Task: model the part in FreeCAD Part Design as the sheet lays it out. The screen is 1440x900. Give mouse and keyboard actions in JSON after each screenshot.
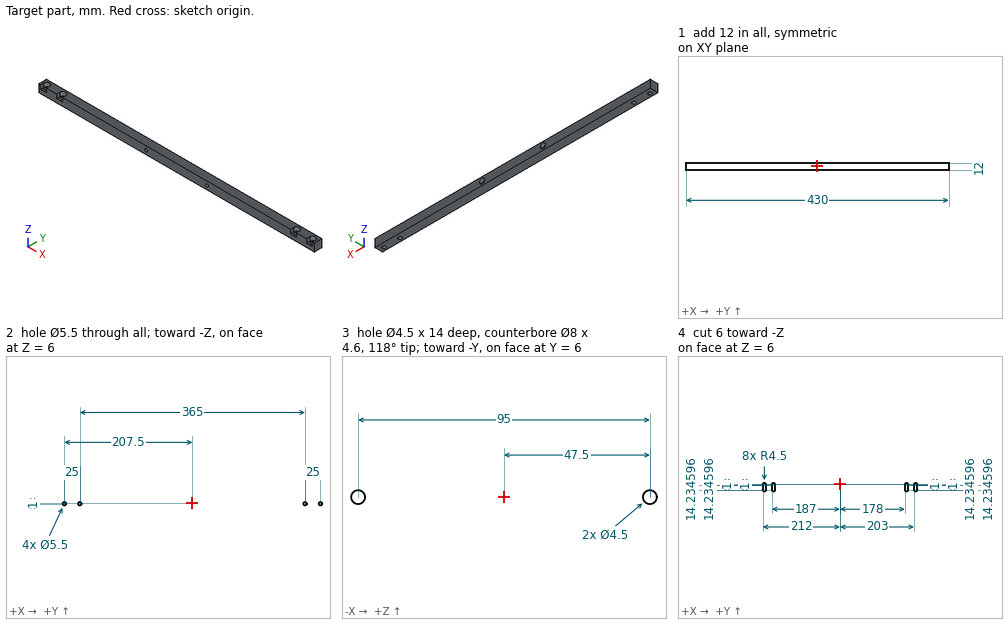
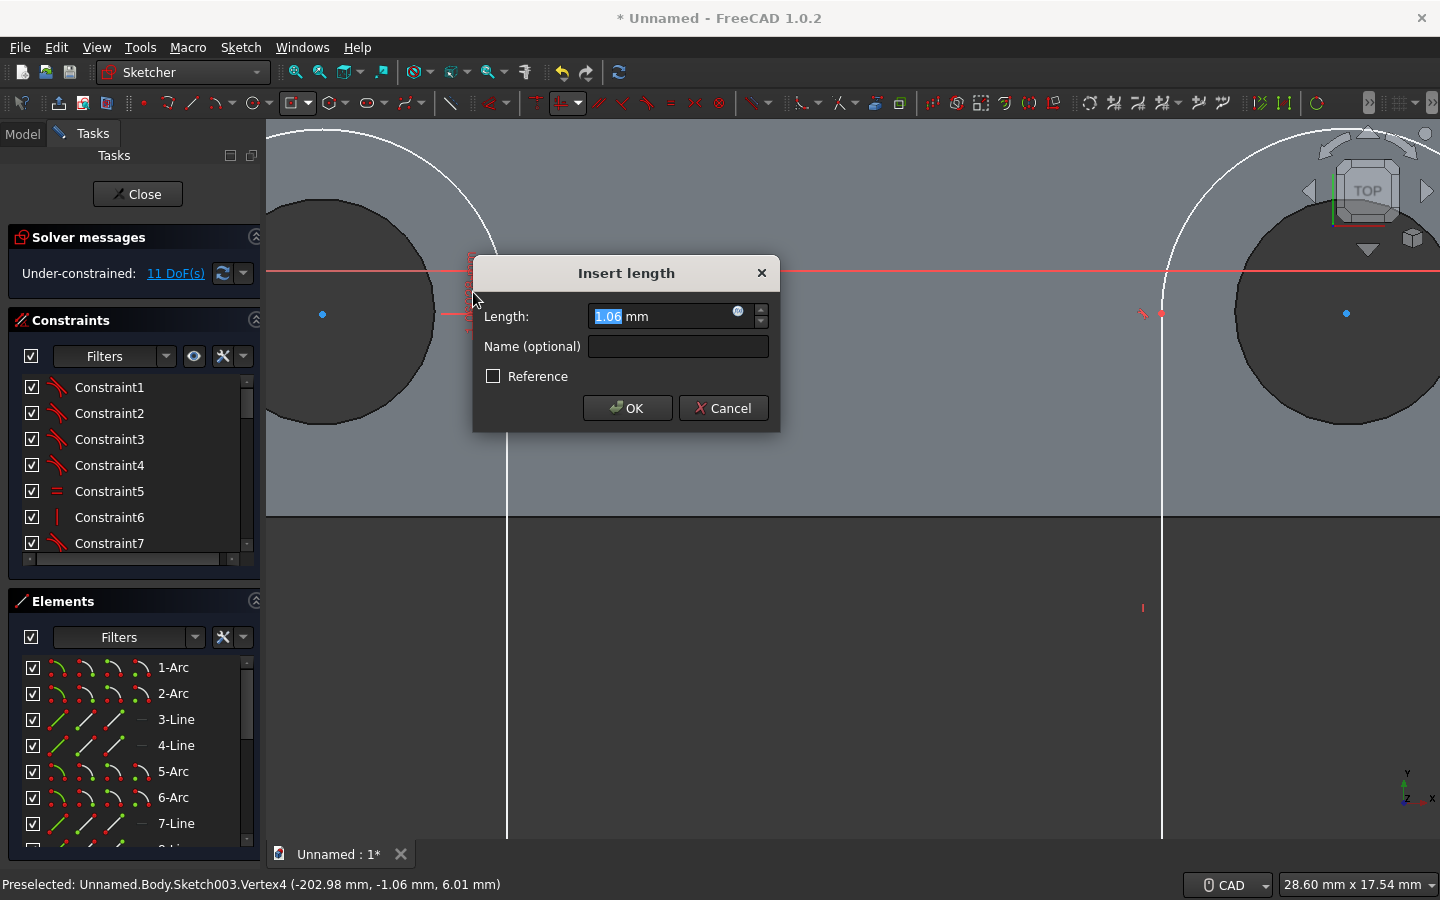
{"action": "type", "text": "1"}
{"action": "key", "text": "Return"}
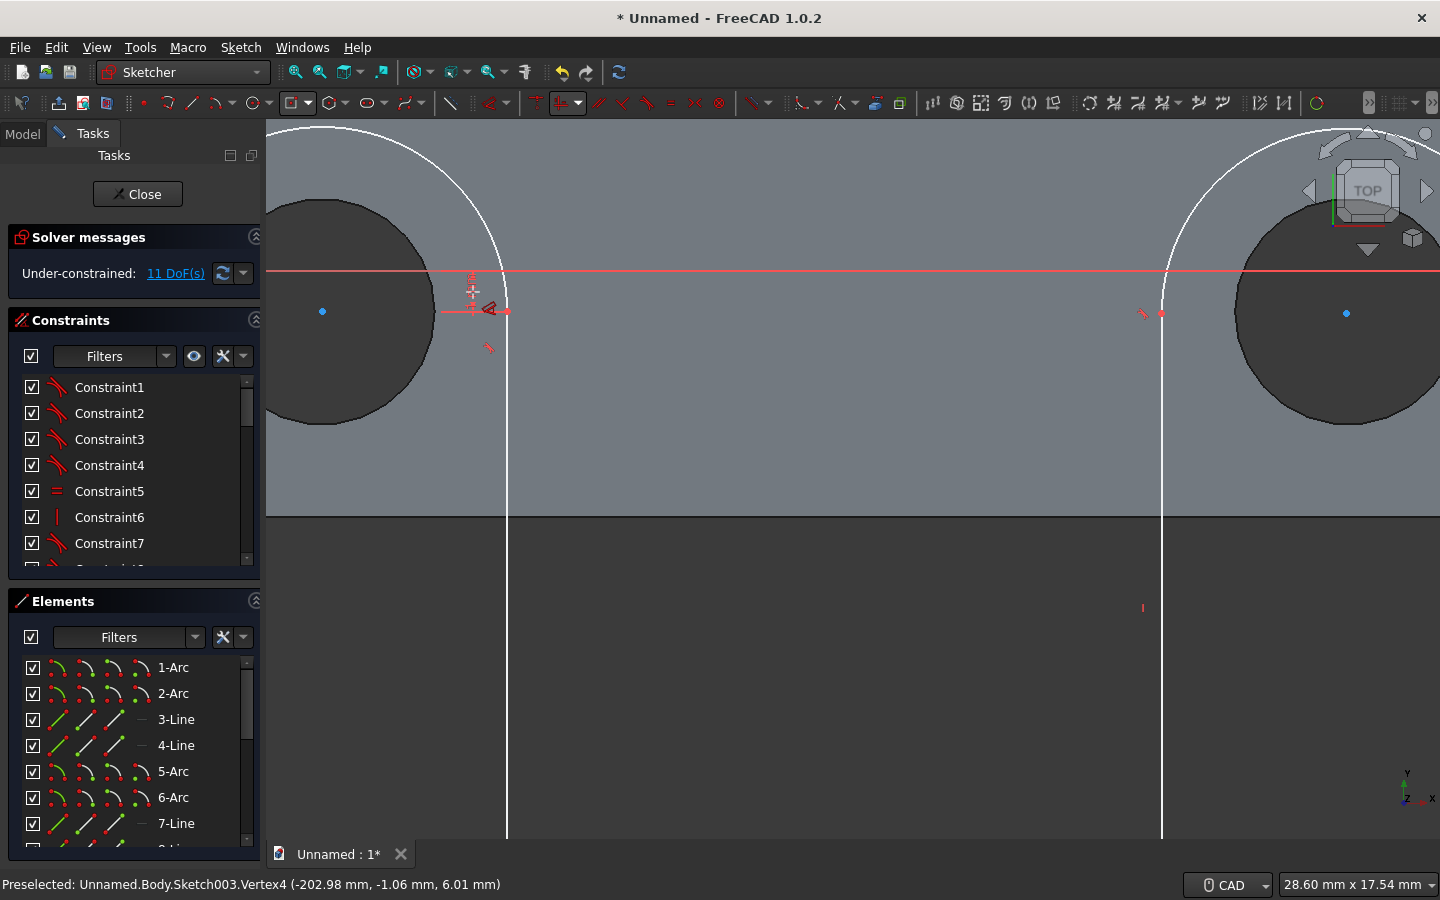
{"action": "scroll", "coordinate": [362, 472], "scroll_direction": "down", "scroll_amount": 15}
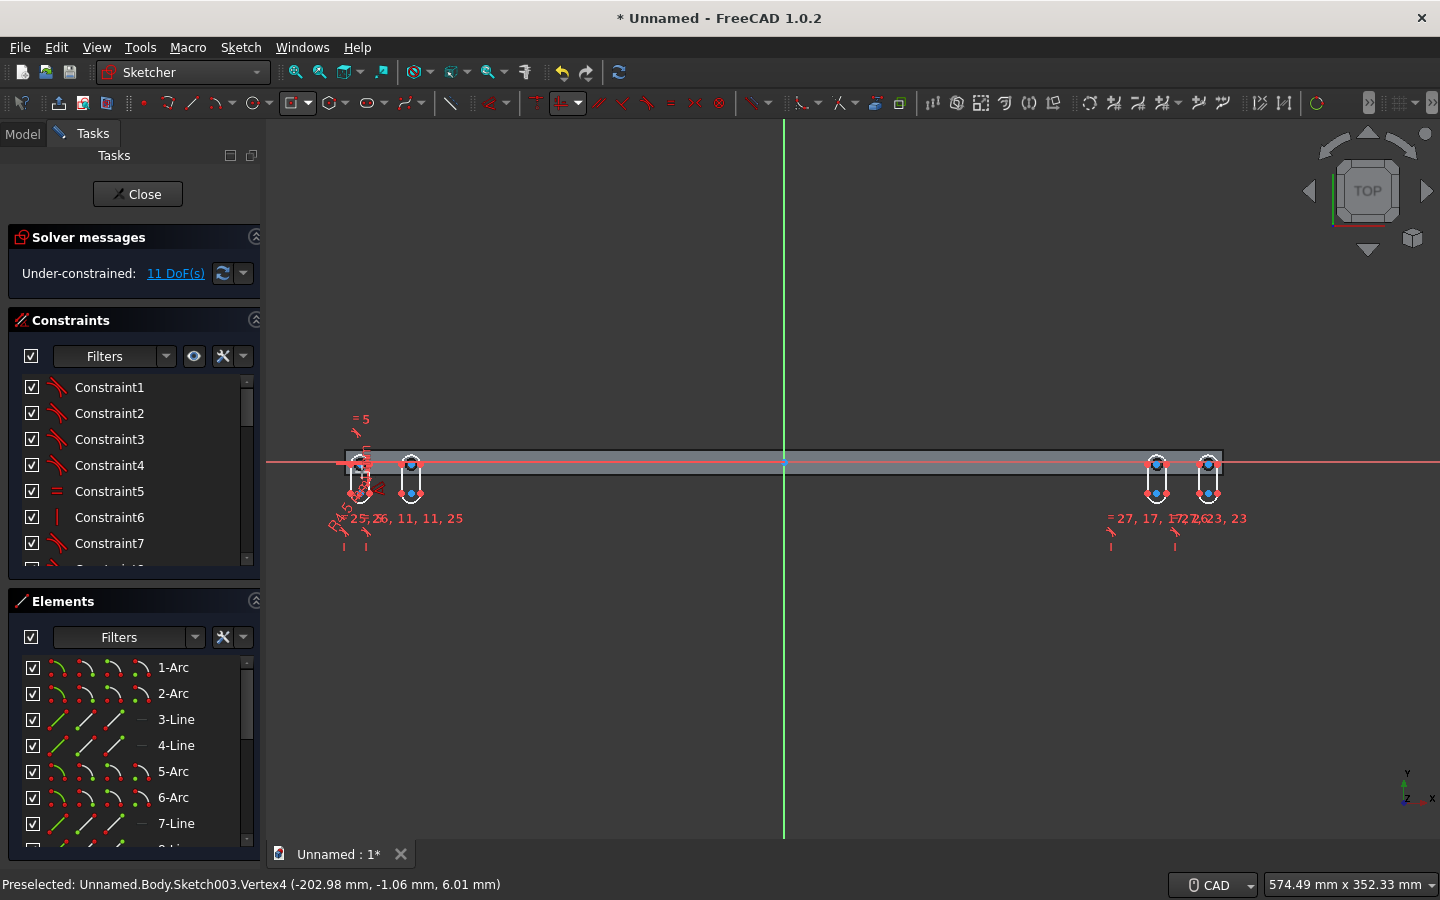
{"action": "scroll", "coordinate": [420, 465], "scroll_direction": "up", "scroll_amount": 15}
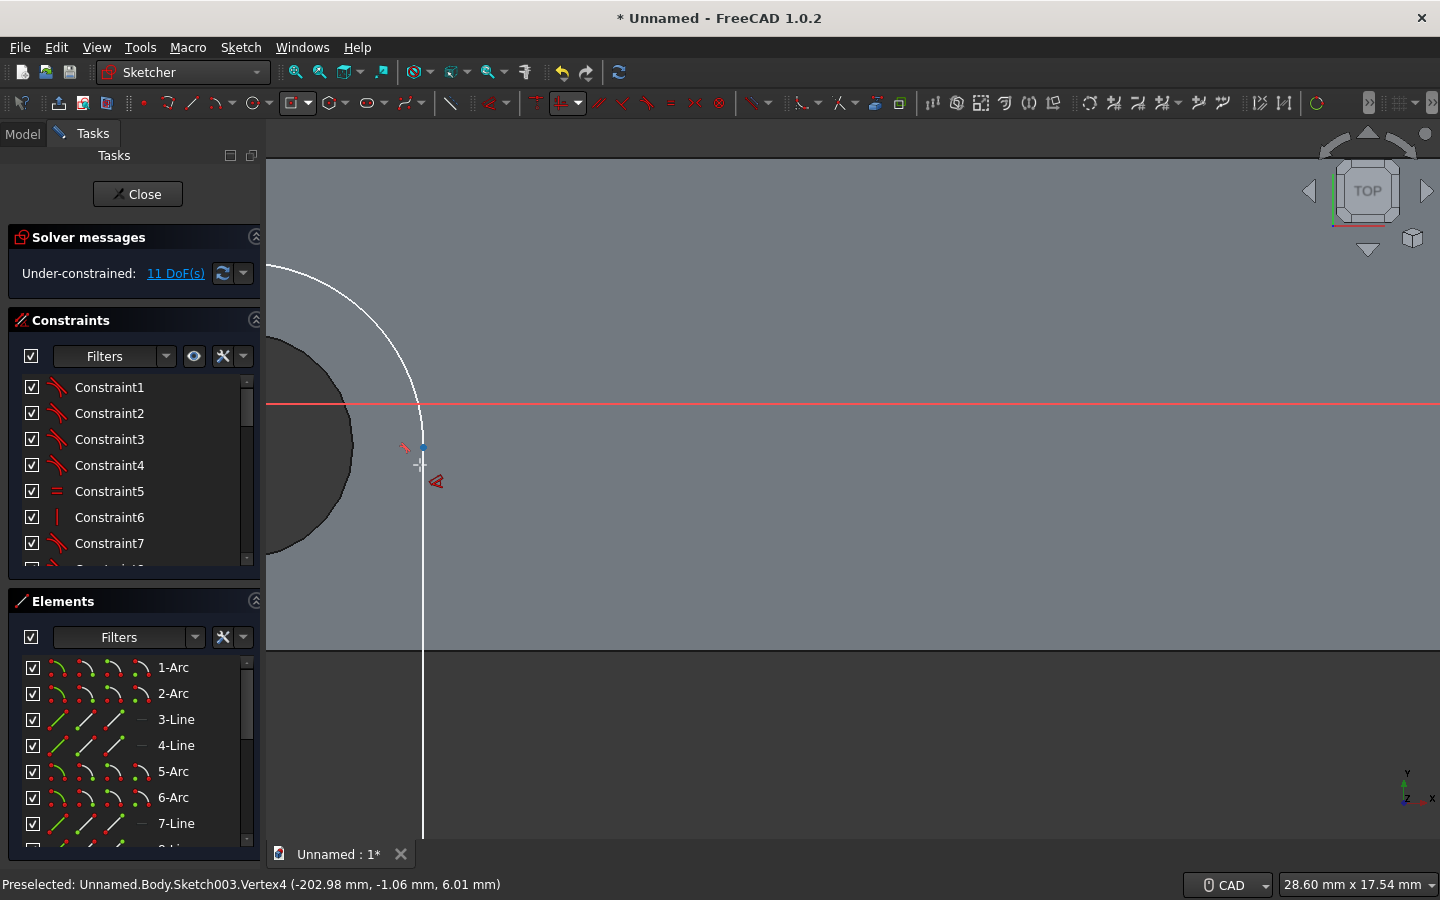
{"action": "left_click", "coordinate": [423, 447]}
{"action": "left_click", "coordinate": [389, 426]}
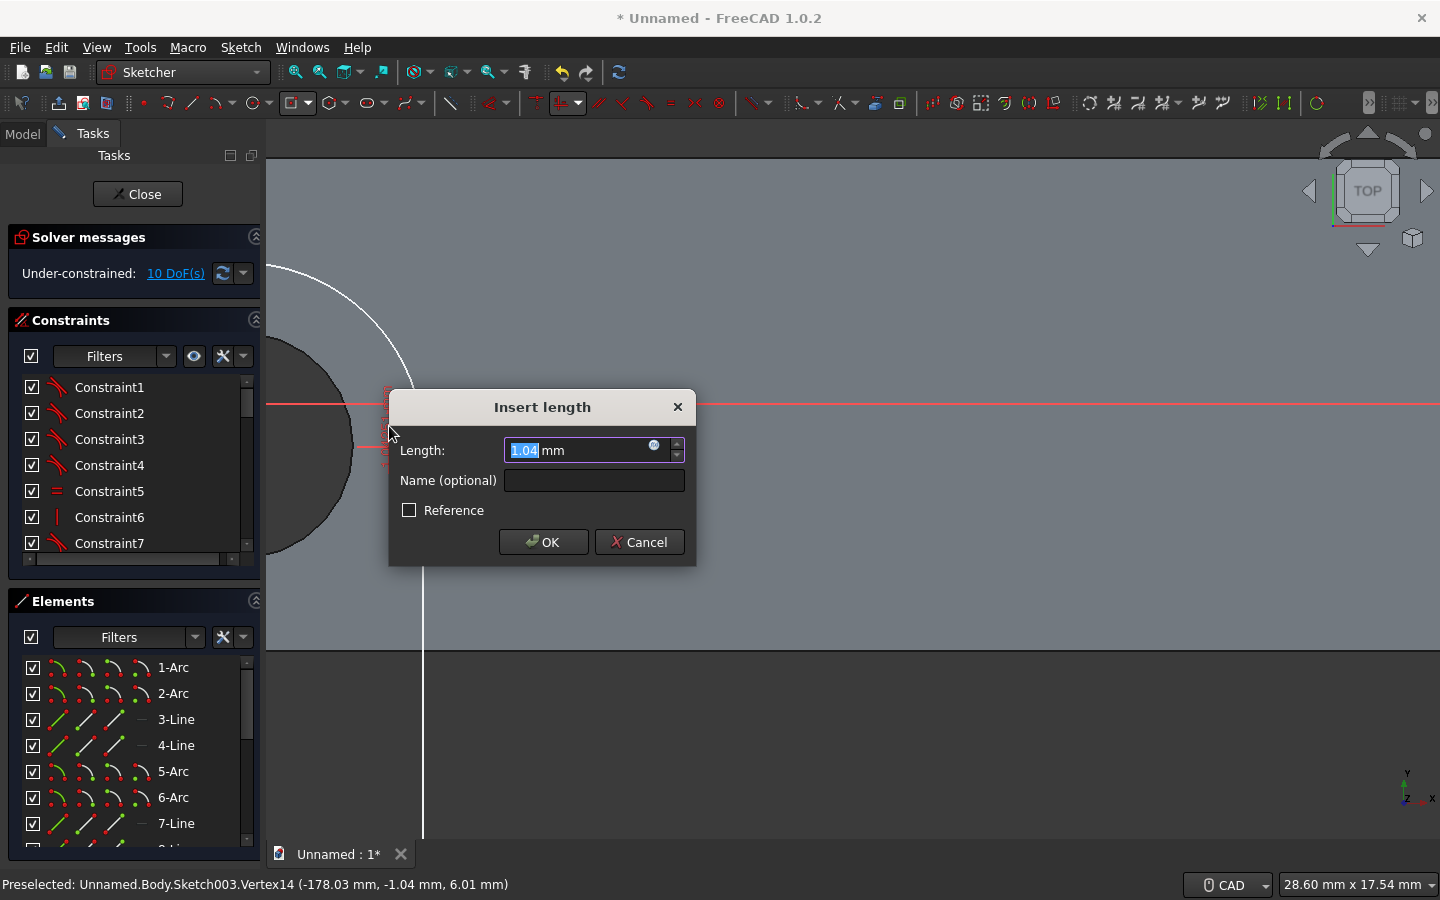
{"action": "type", "text": "1"}
{"action": "key", "text": "Return"}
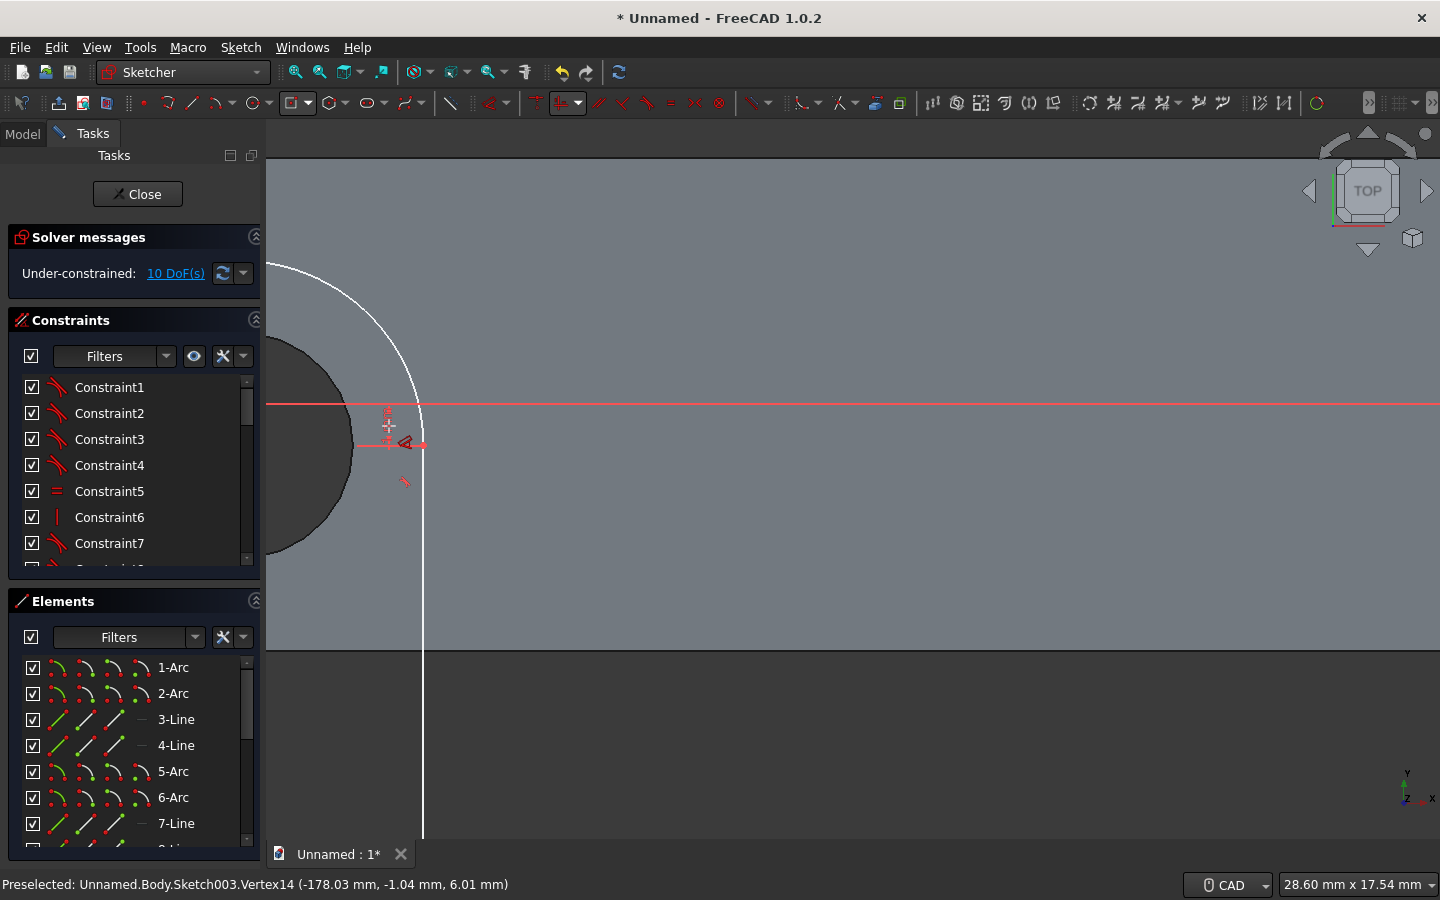
{"action": "scroll", "coordinate": [421, 465], "scroll_direction": "down", "scroll_amount": 15}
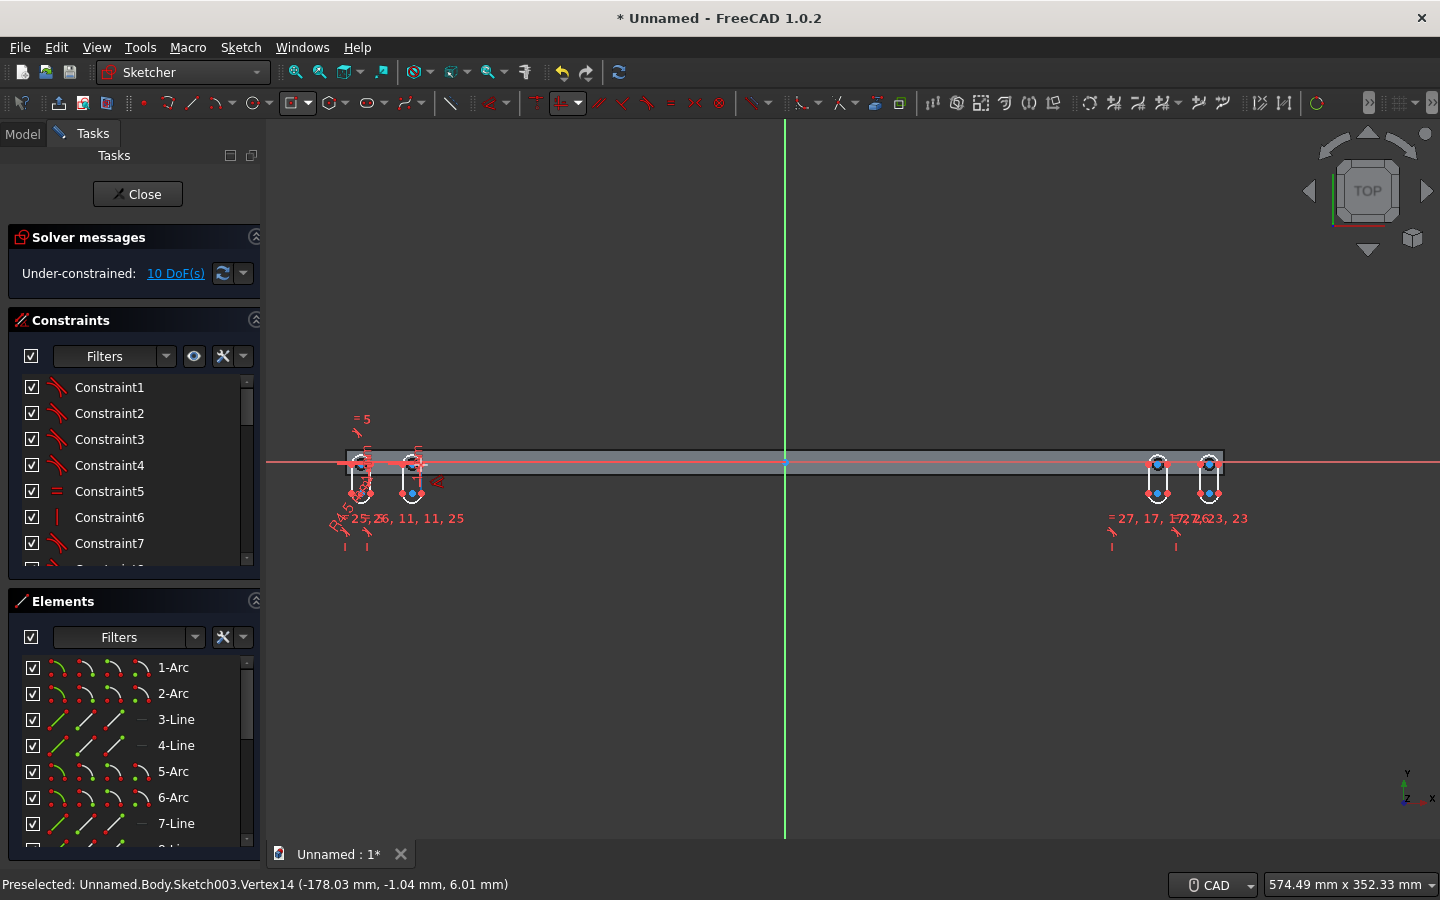
{"action": "scroll", "coordinate": [1167, 465], "scroll_direction": "up", "scroll_amount": 15}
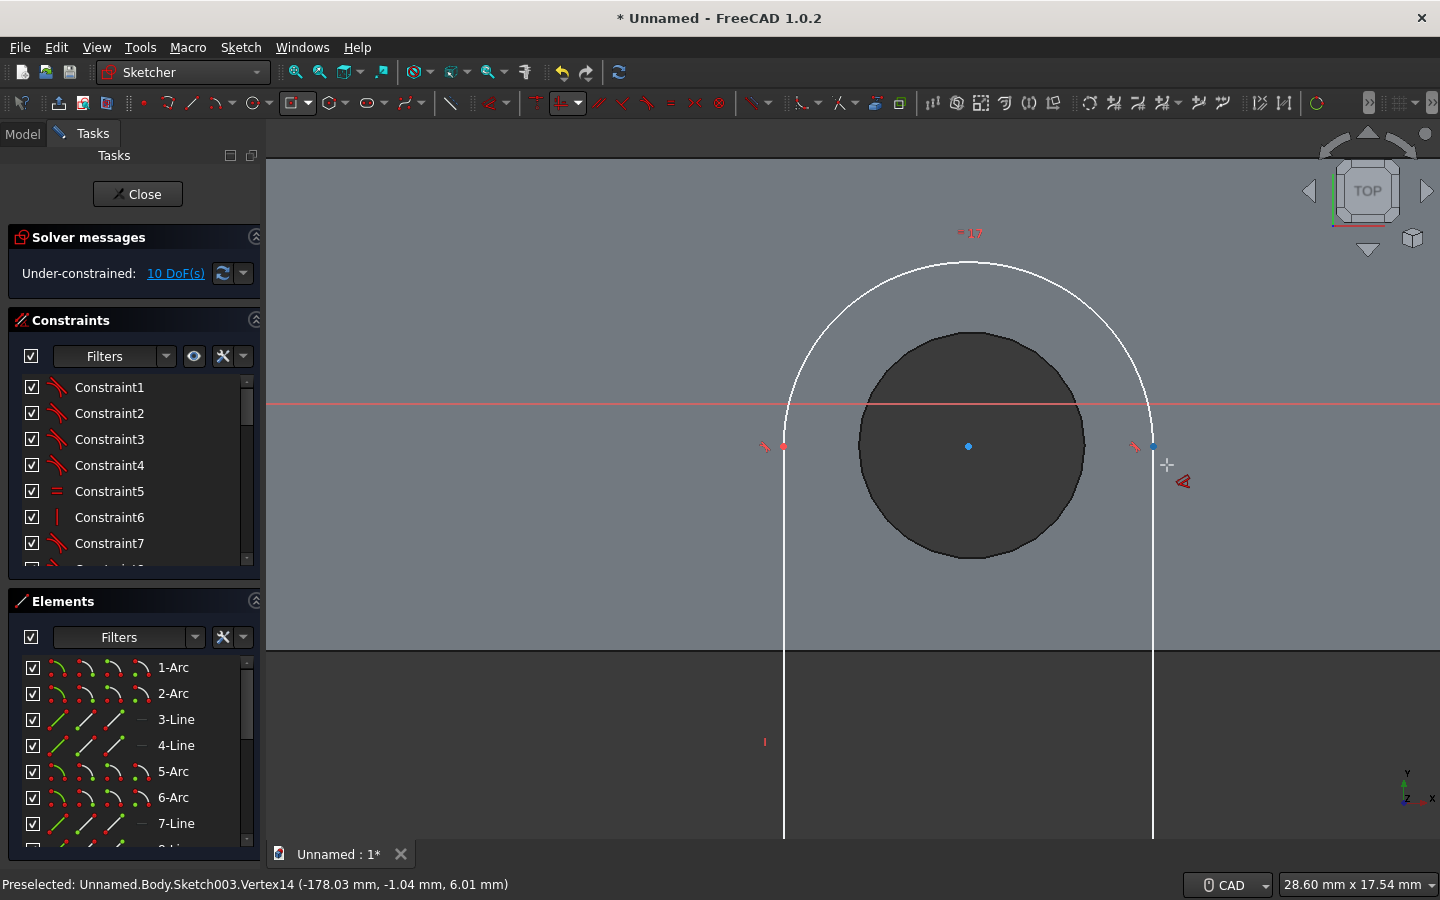
{"action": "left_click", "coordinate": [1153, 447]}
{"action": "left_click", "coordinate": [1187, 426]}